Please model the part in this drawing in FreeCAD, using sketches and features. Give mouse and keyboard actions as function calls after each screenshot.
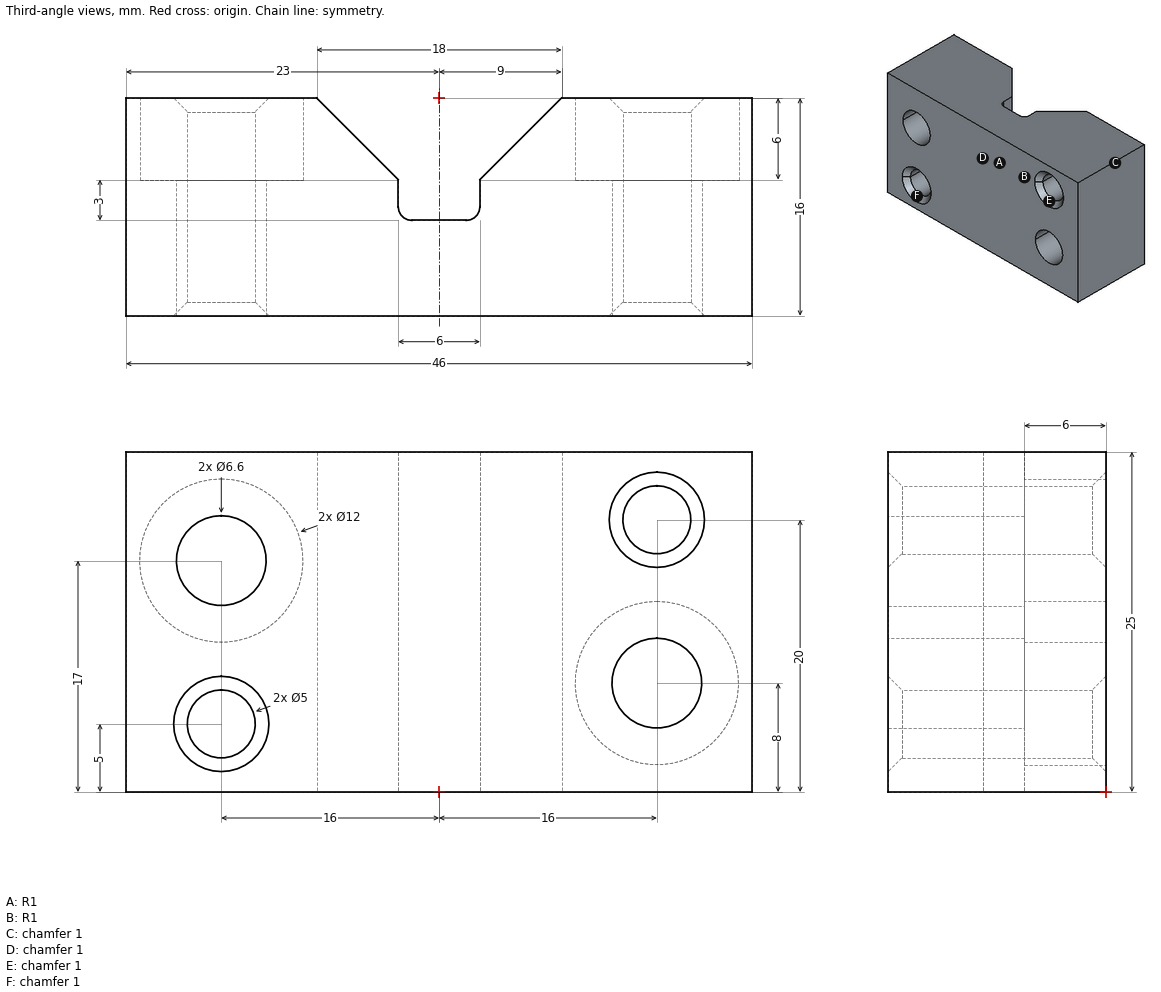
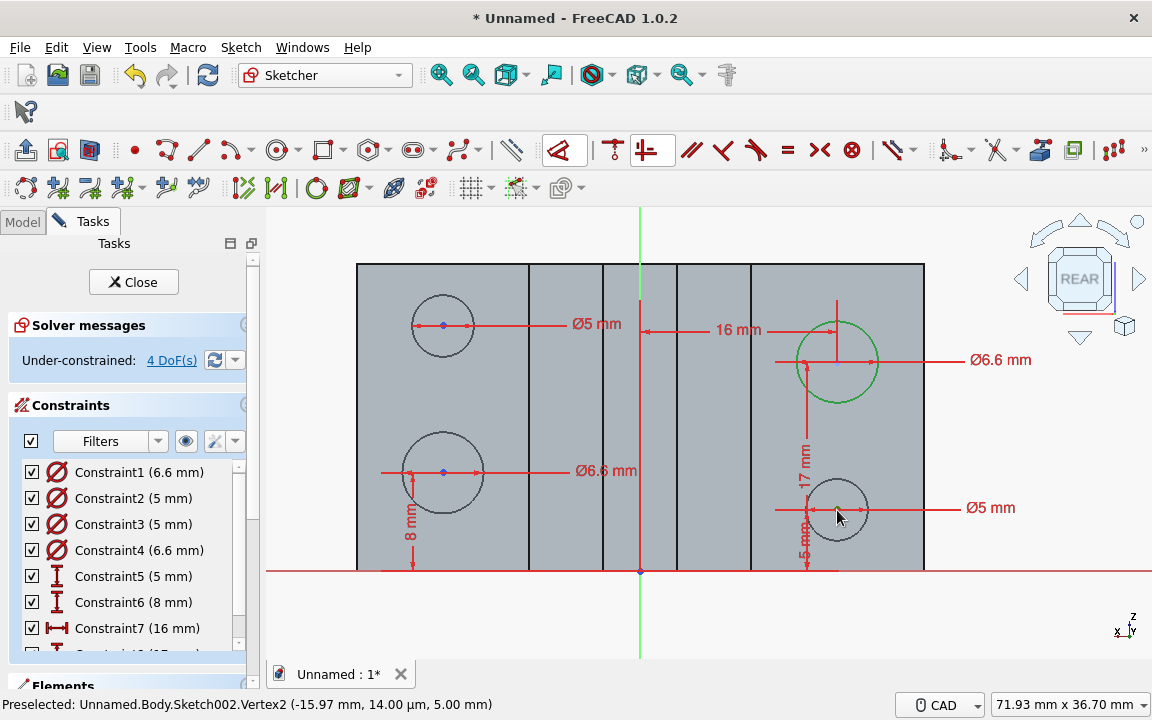
click(582, 150)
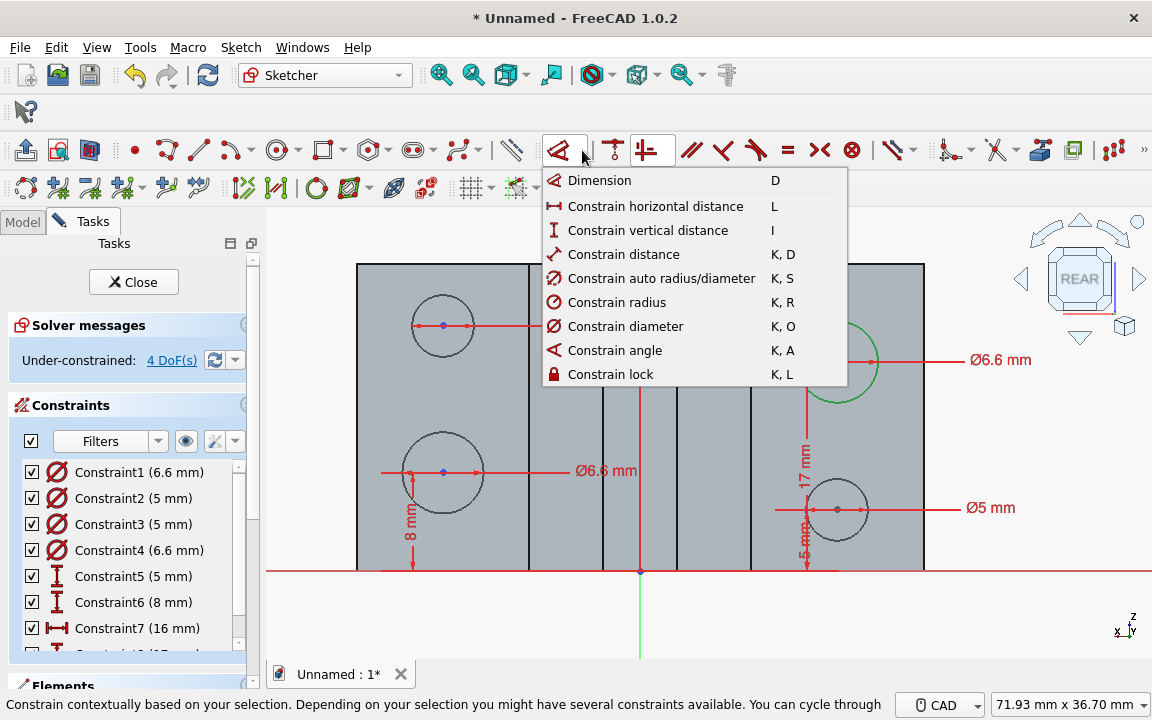
click(695, 206)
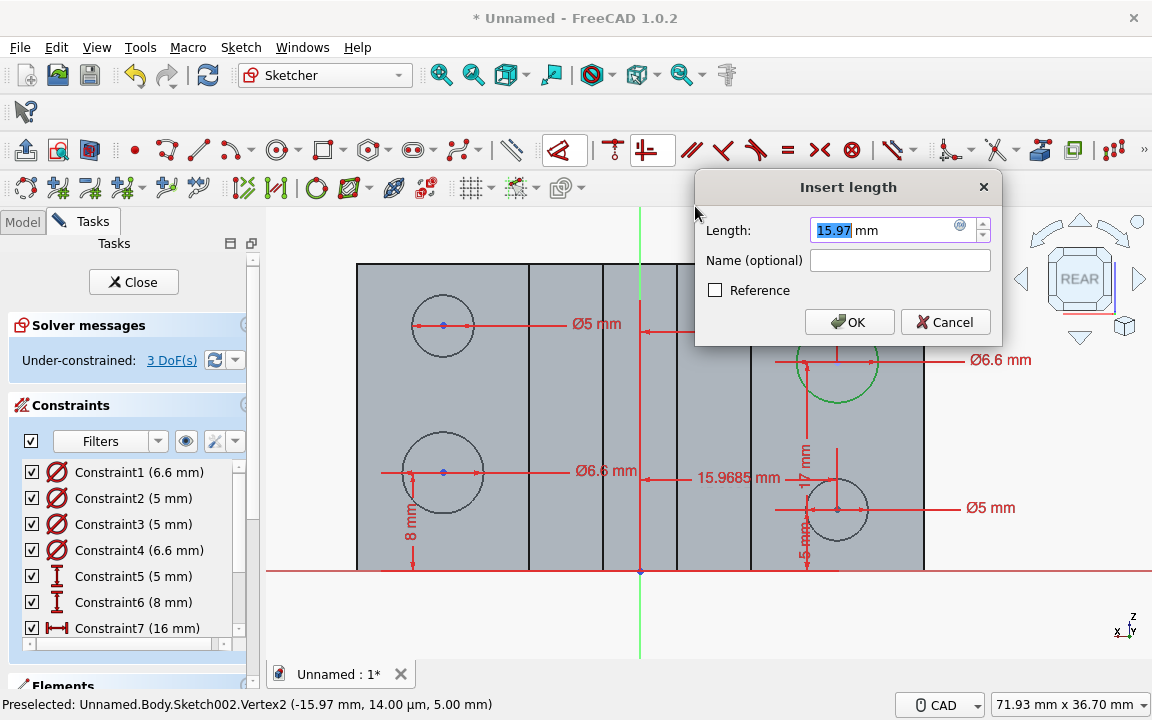
text(16)
key(Return)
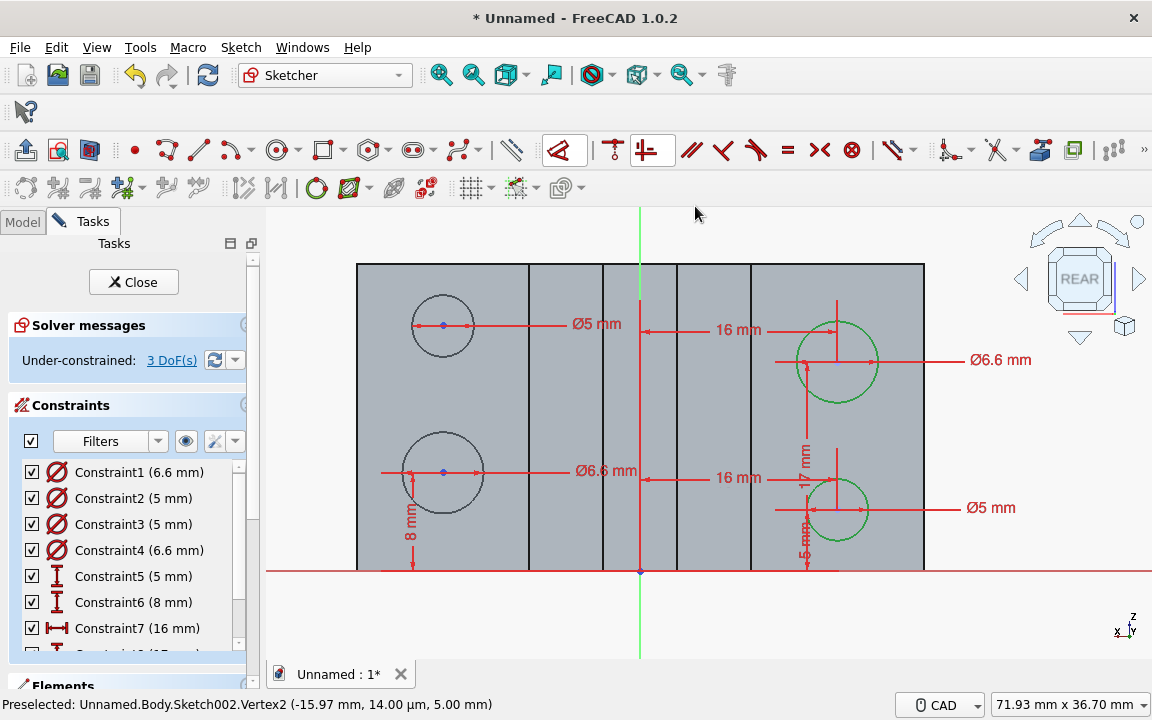
click(443, 326)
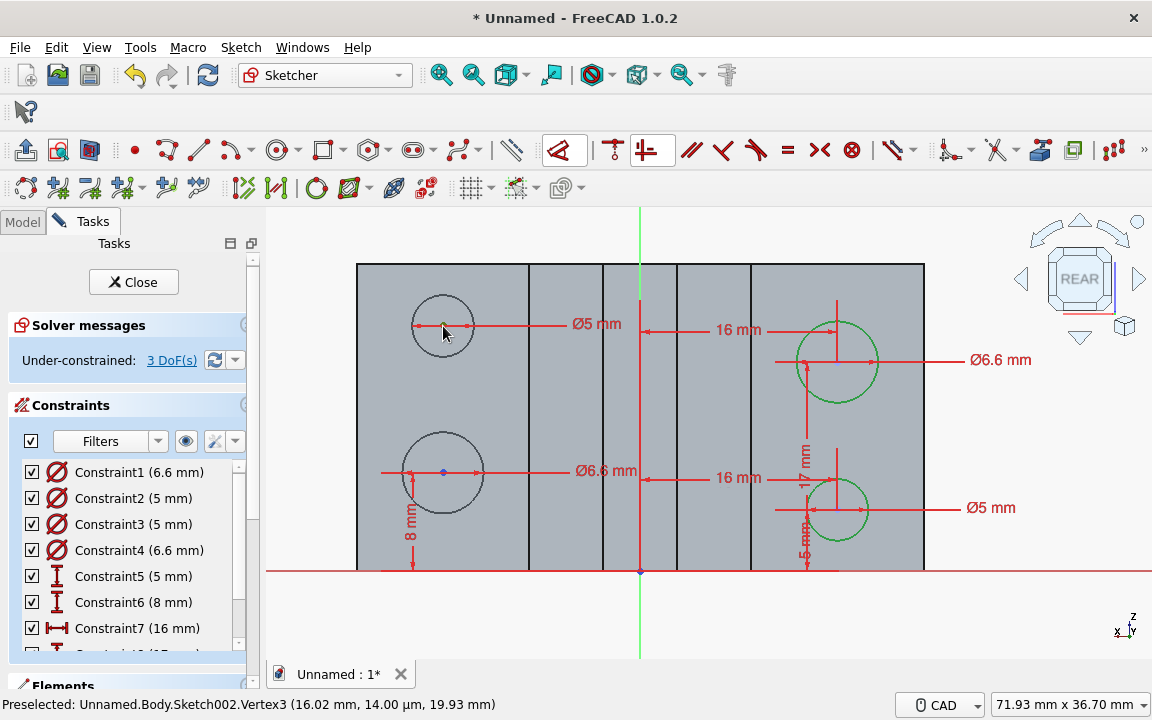
click(582, 150)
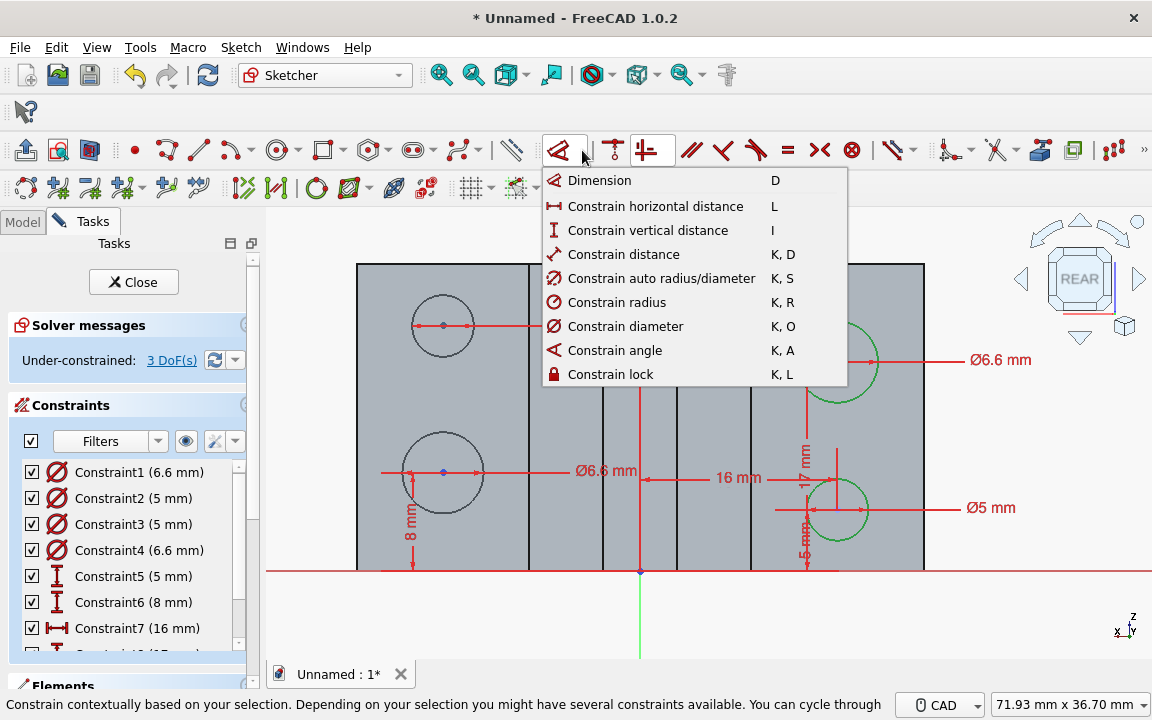
click(695, 206)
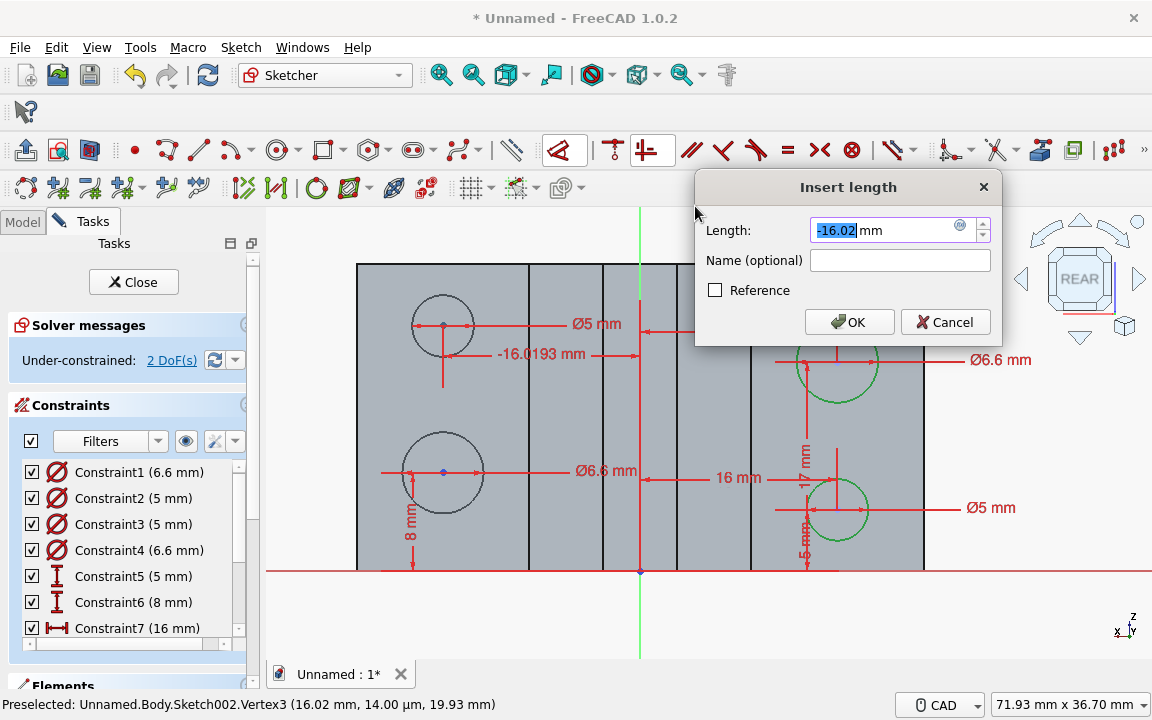
text(-16)
key(Return)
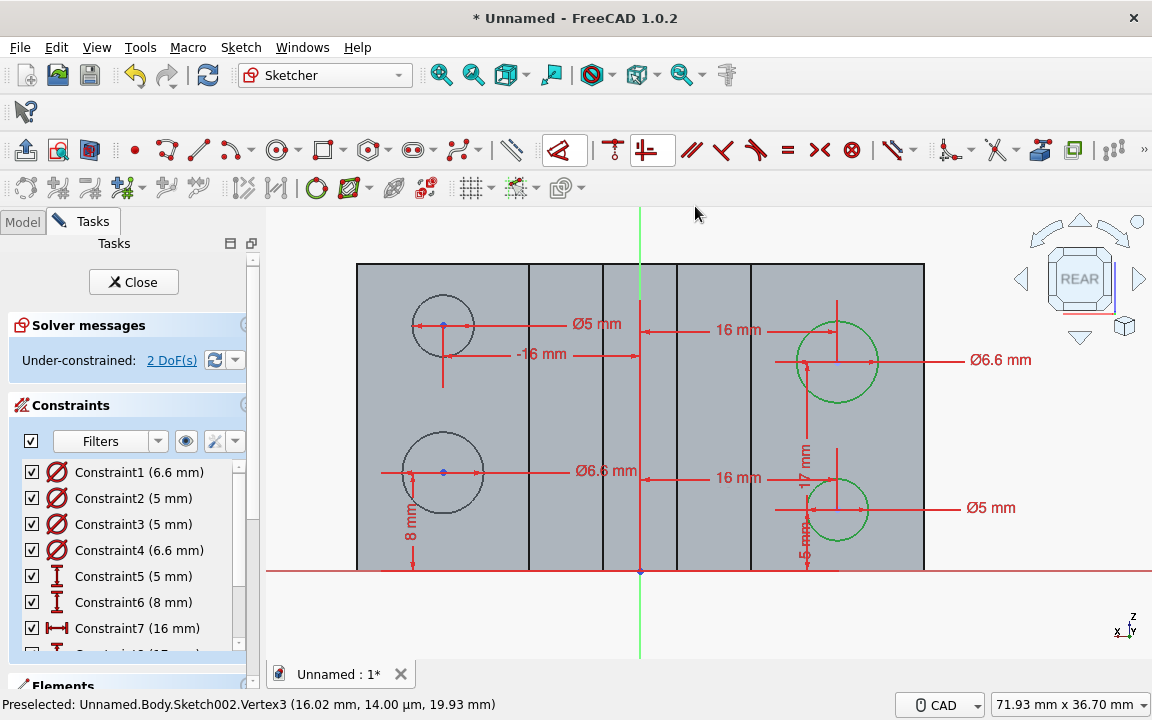
click(443, 326)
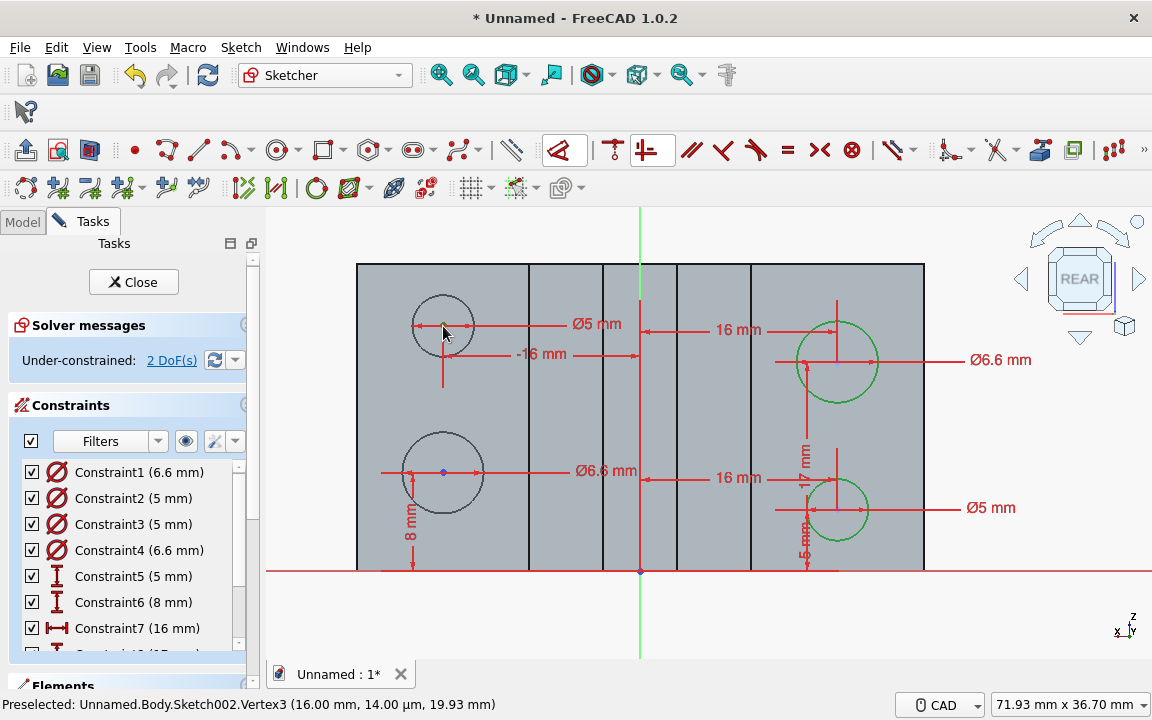
click(582, 150)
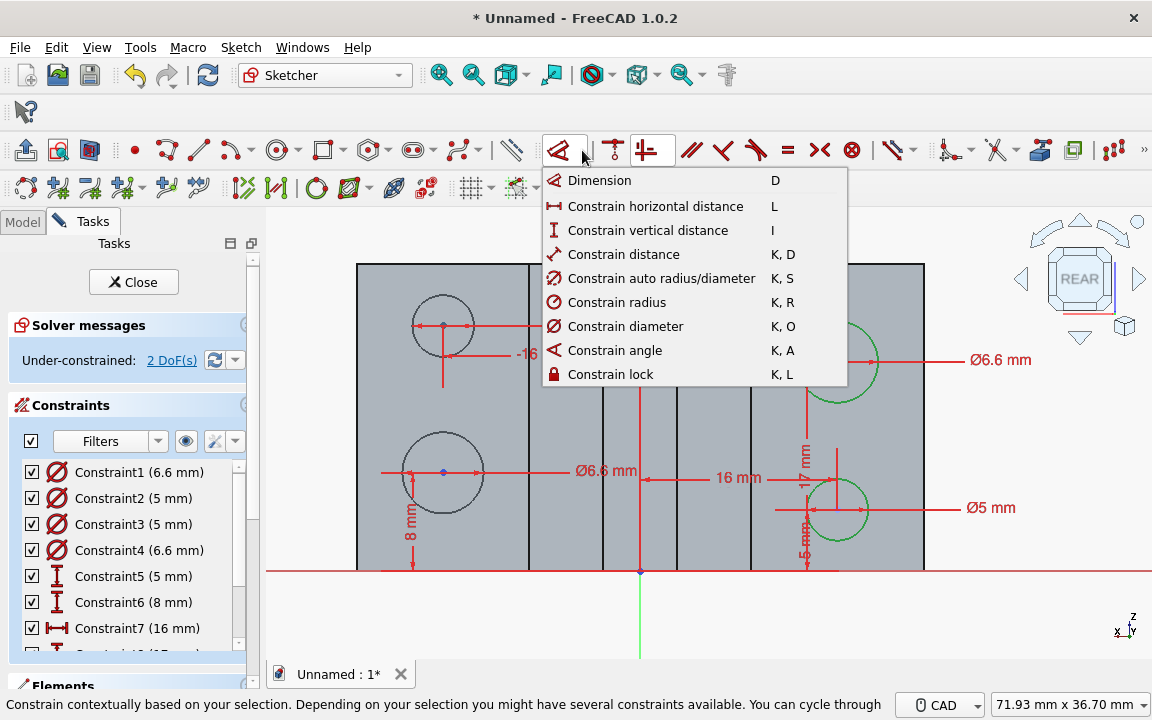
click(695, 230)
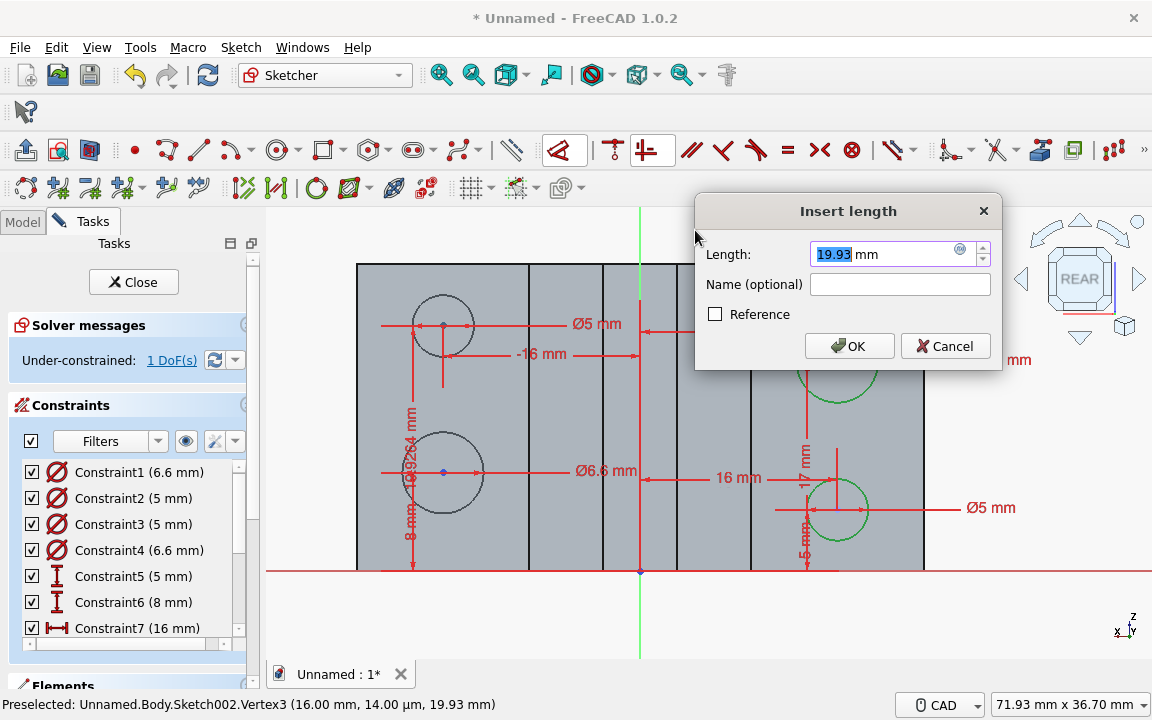
text(20)
key(Return)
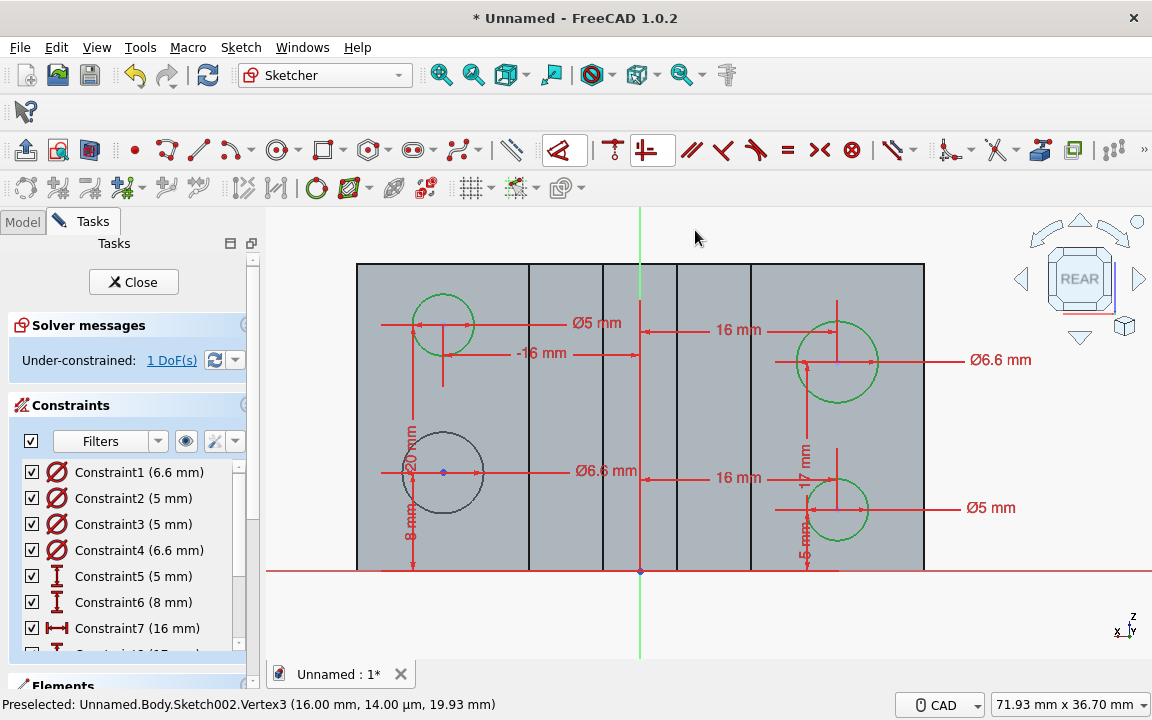
click(443, 473)